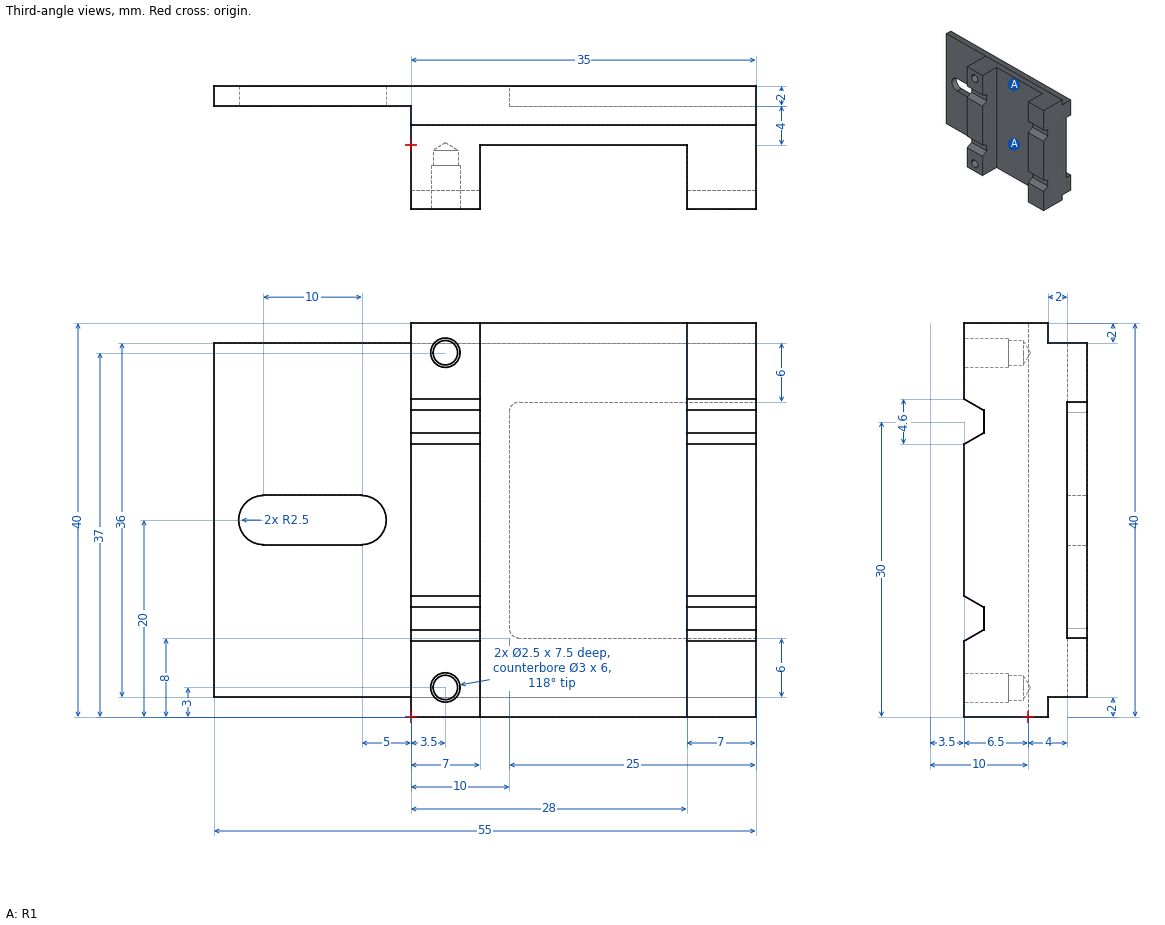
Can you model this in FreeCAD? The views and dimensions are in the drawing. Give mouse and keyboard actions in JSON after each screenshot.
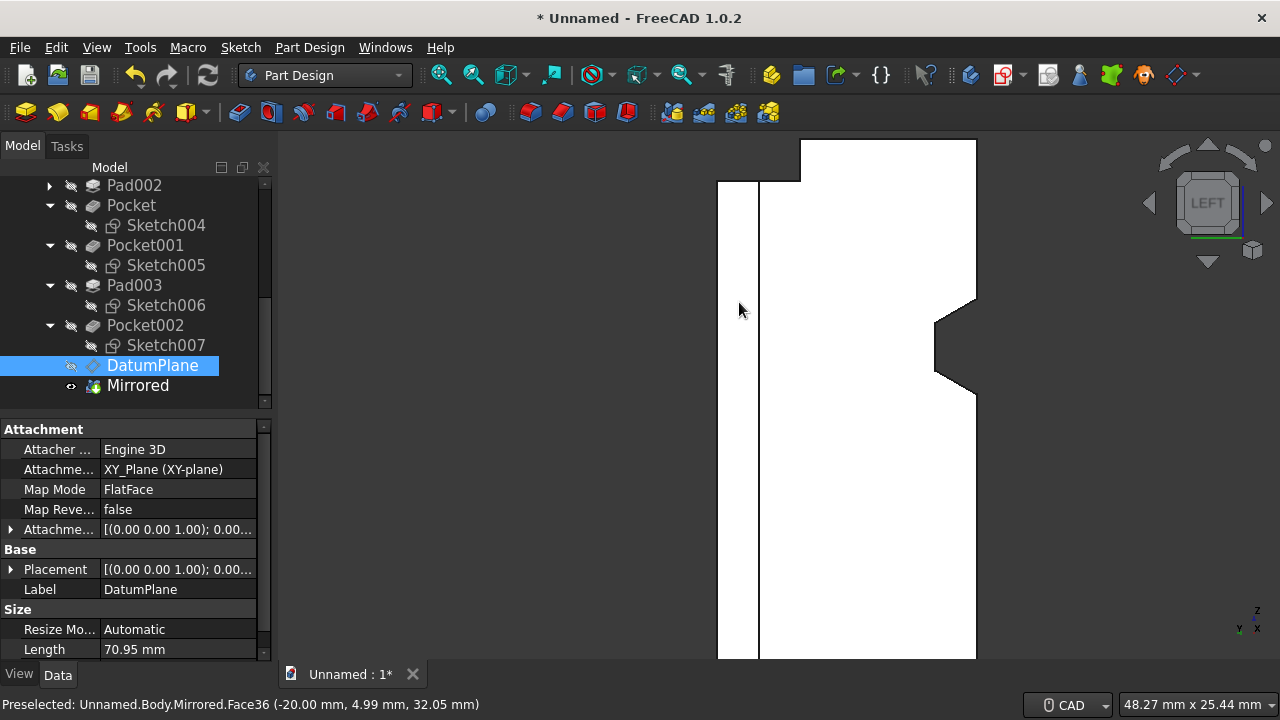
{"action": "left_click", "coordinate": [442, 76]}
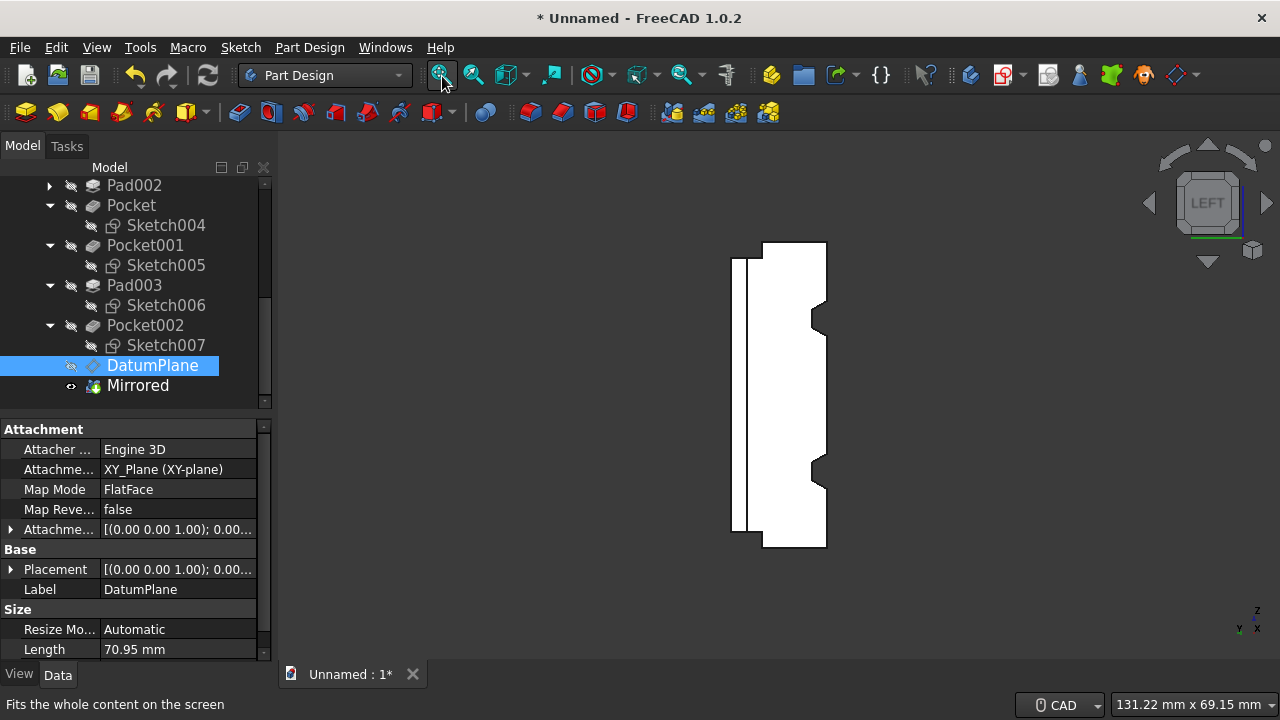
{"action": "key", "text": "v 3"}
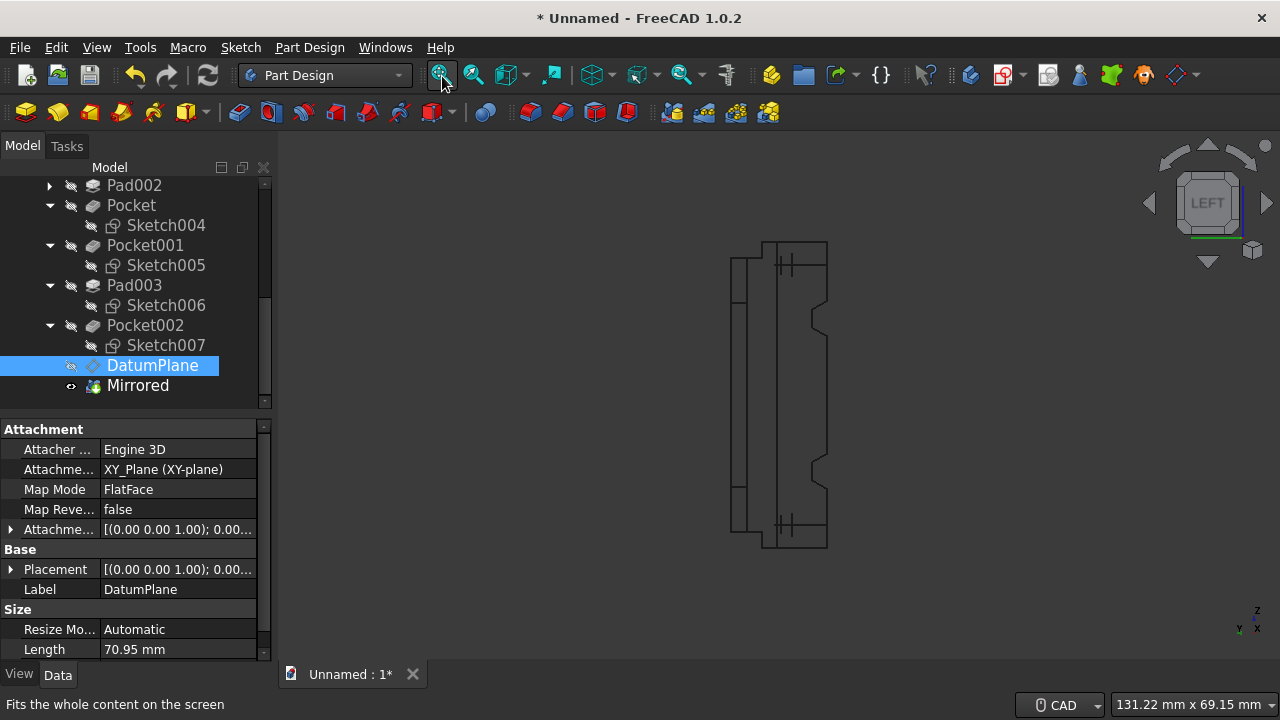
{"action": "key", "text": "0"}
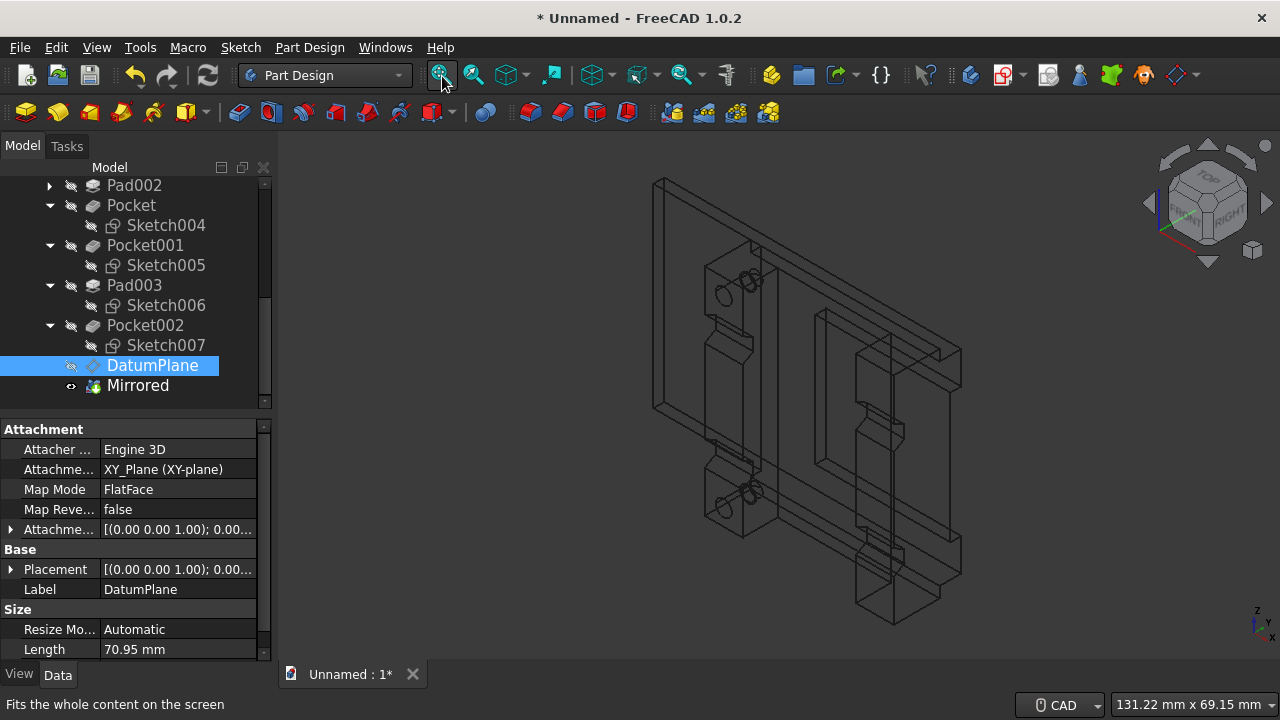
{"action": "left_click", "coordinate": [822, 310]}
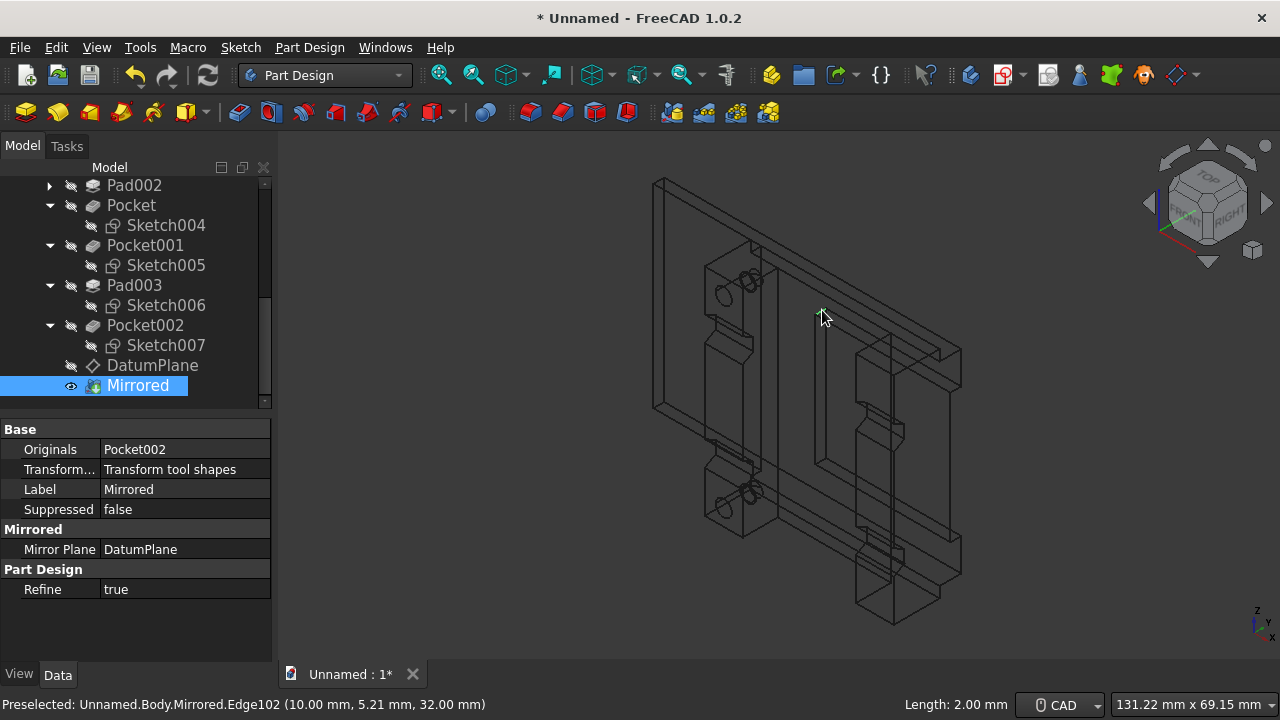
{"action": "left_click", "coordinate": [823, 459], "text": "ctrl"}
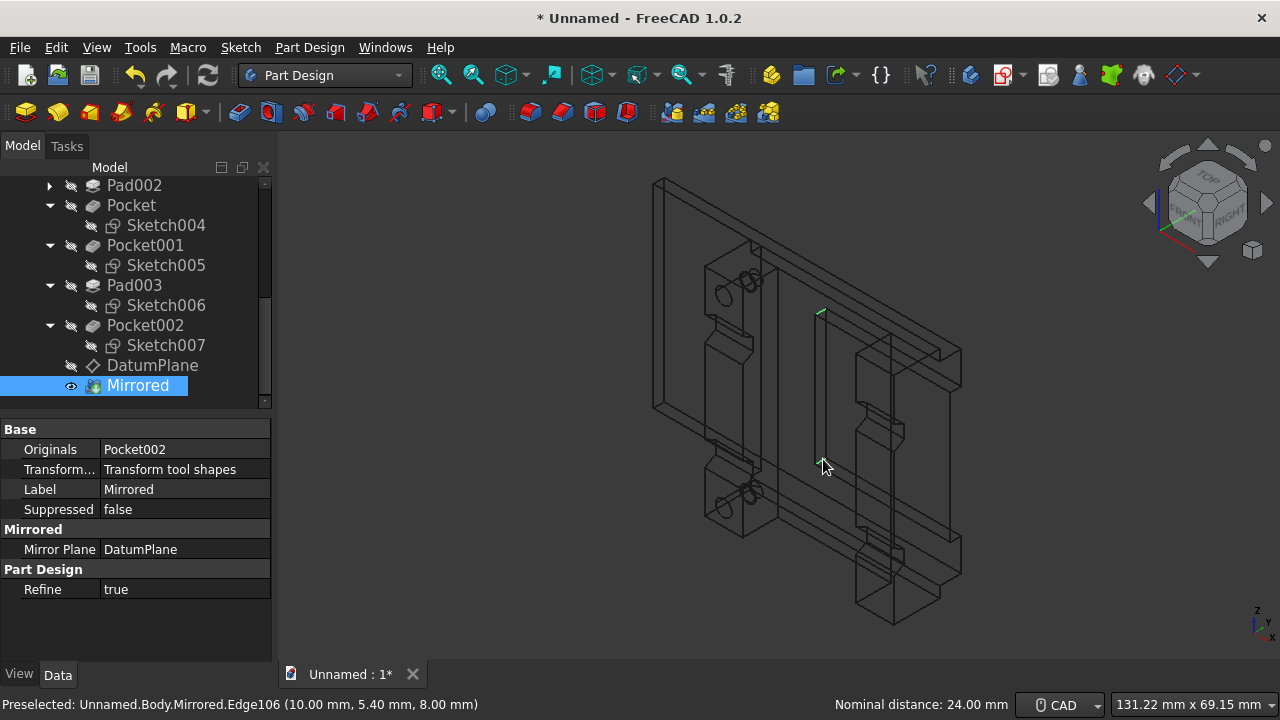
{"action": "key", "text": "v 1"}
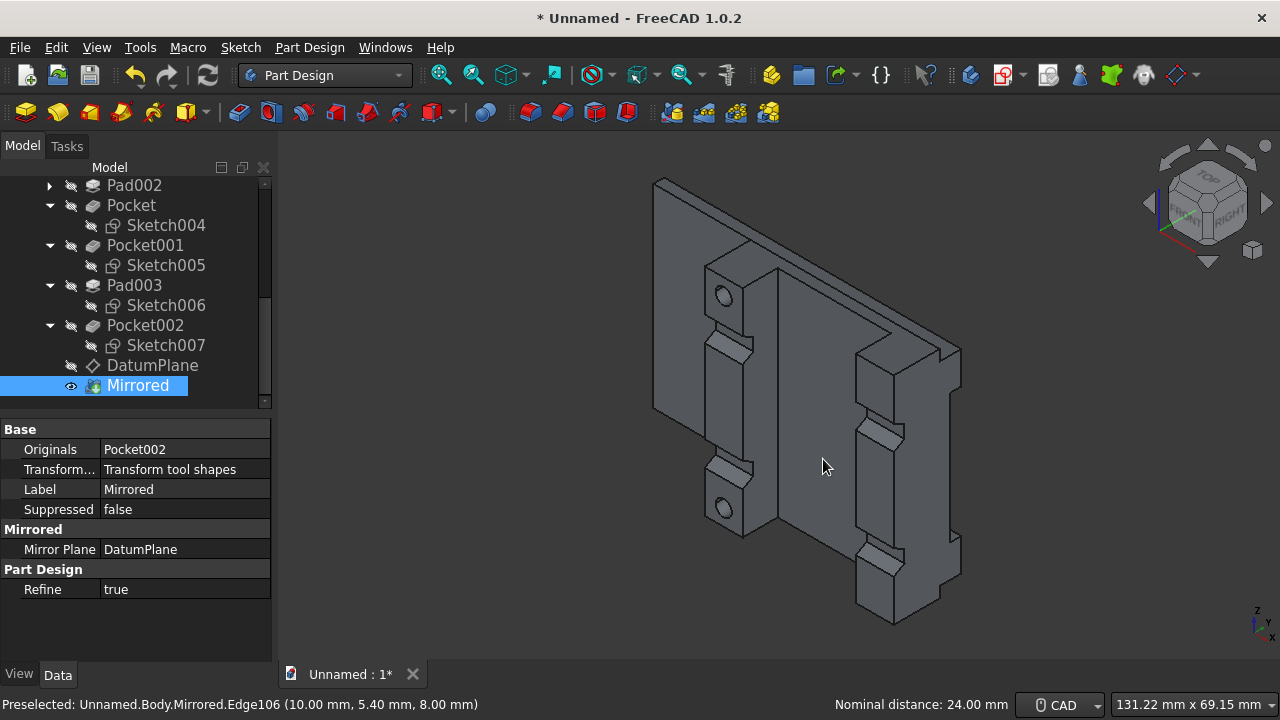
{"action": "left_click", "coordinate": [532, 112]}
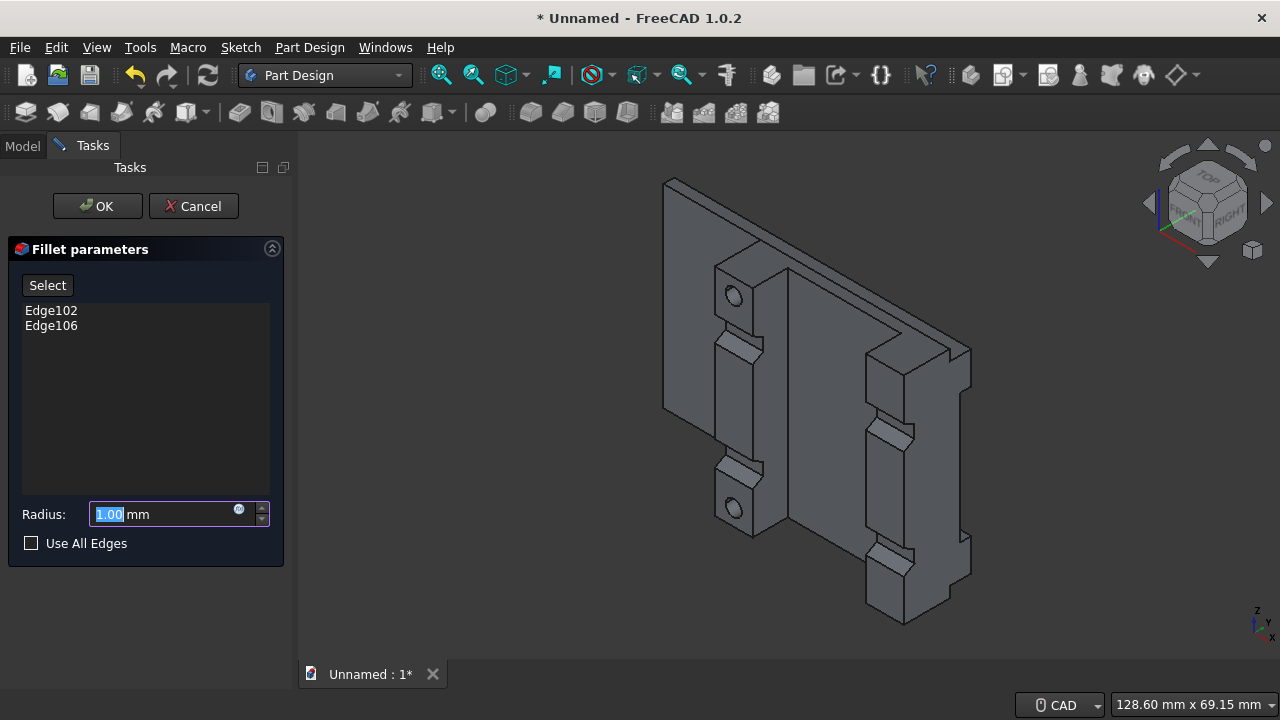
{"action": "type", "text": "1"}
{"action": "key", "text": "Tab"}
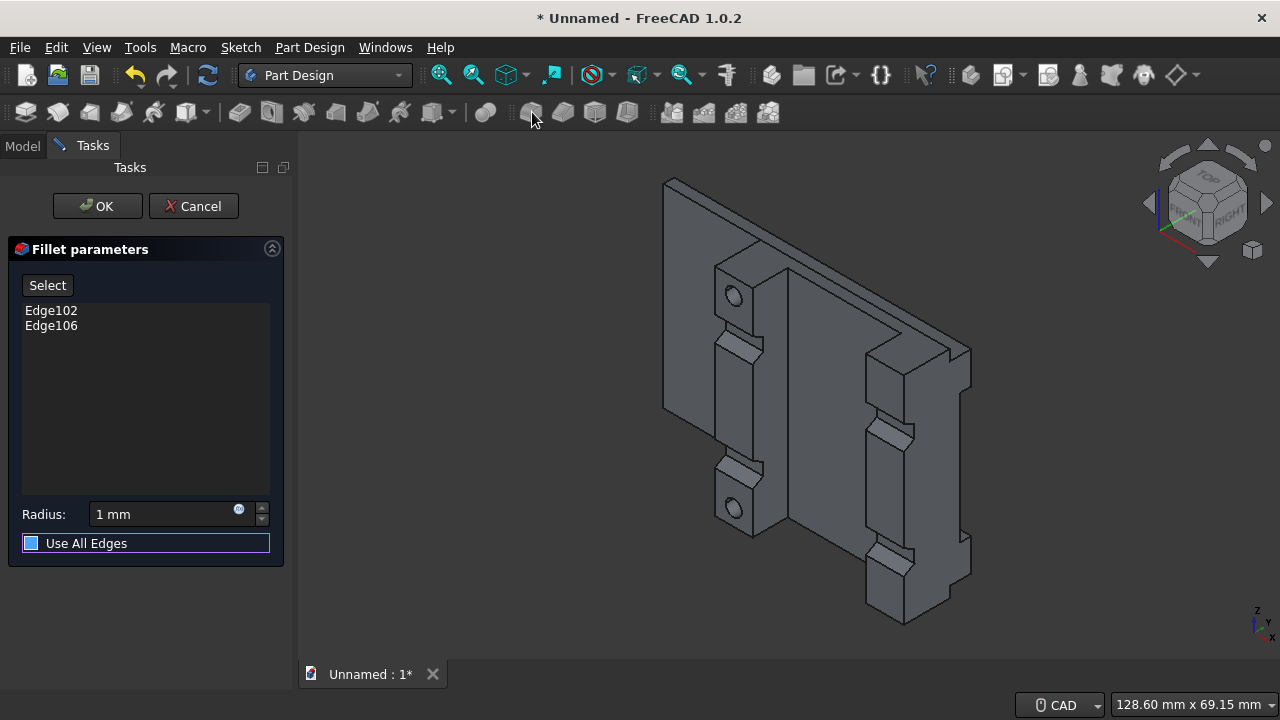
{"action": "left_click", "coordinate": [98, 206]}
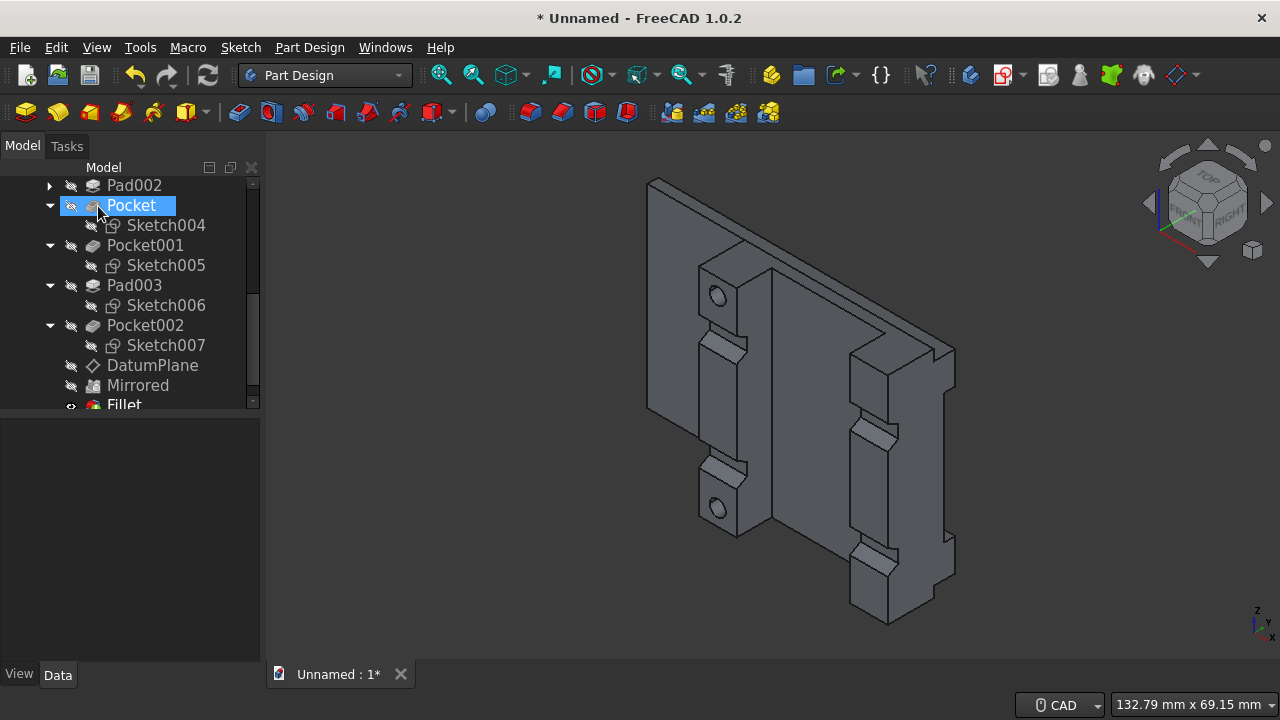
{"action": "left_click", "coordinate": [686, 253]}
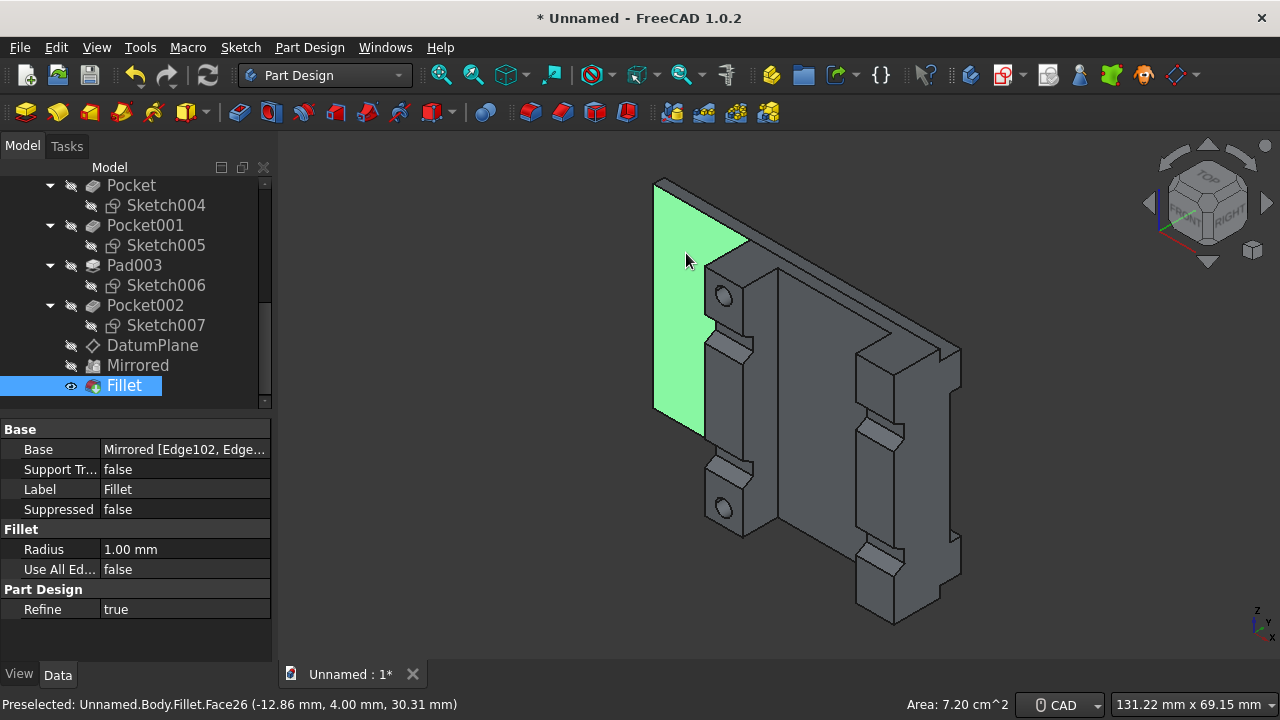
{"action": "left_click", "coordinate": [1004, 76]}